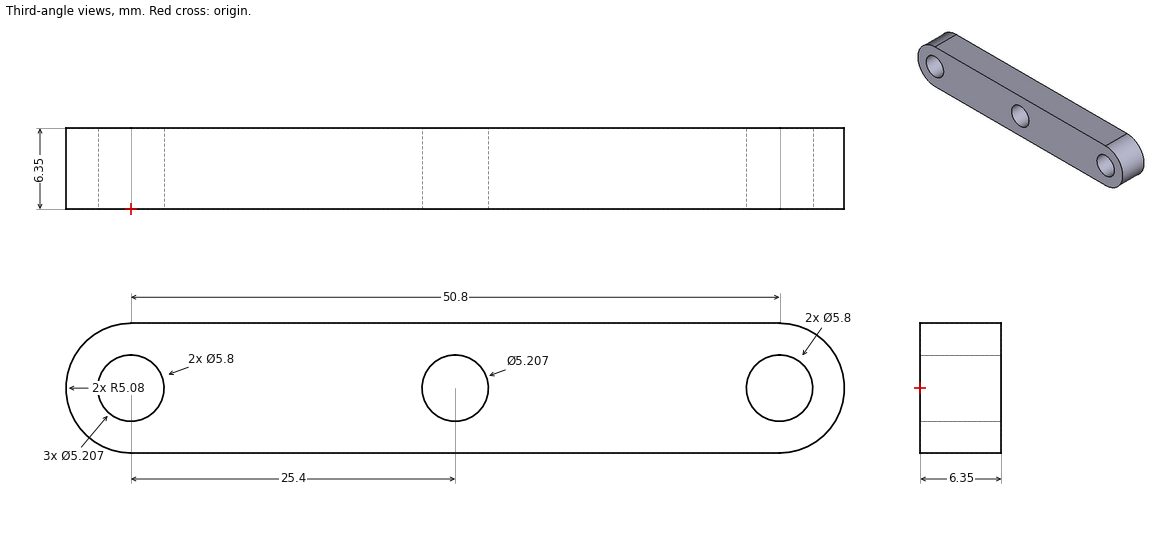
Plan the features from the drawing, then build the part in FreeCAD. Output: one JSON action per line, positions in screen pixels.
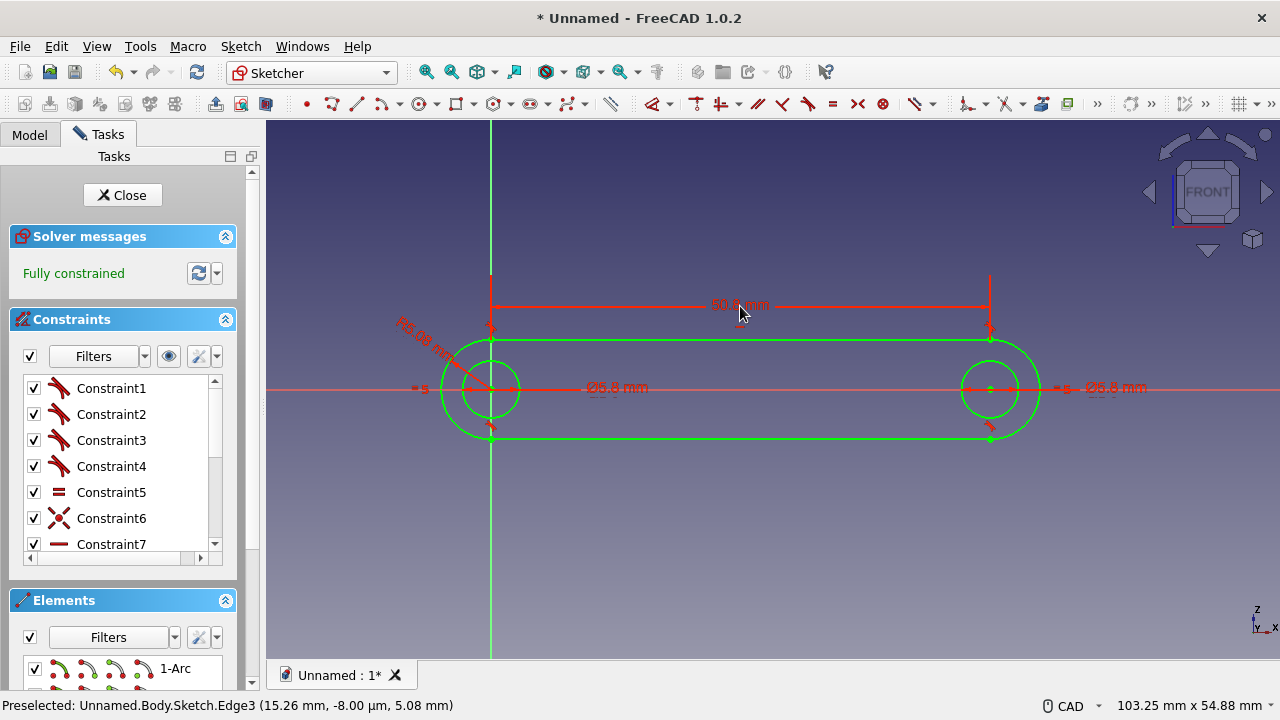
{"action": "left_click", "coordinate": [123, 195]}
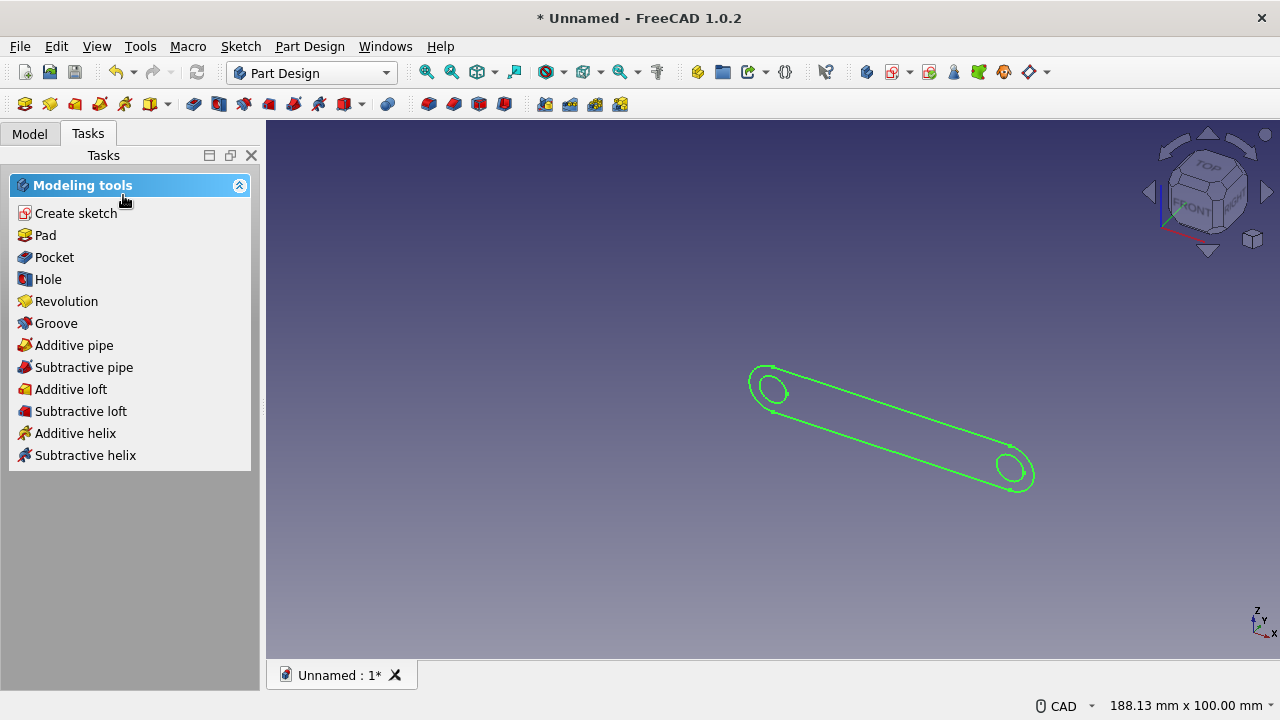
{"action": "left_click", "coordinate": [25, 104]}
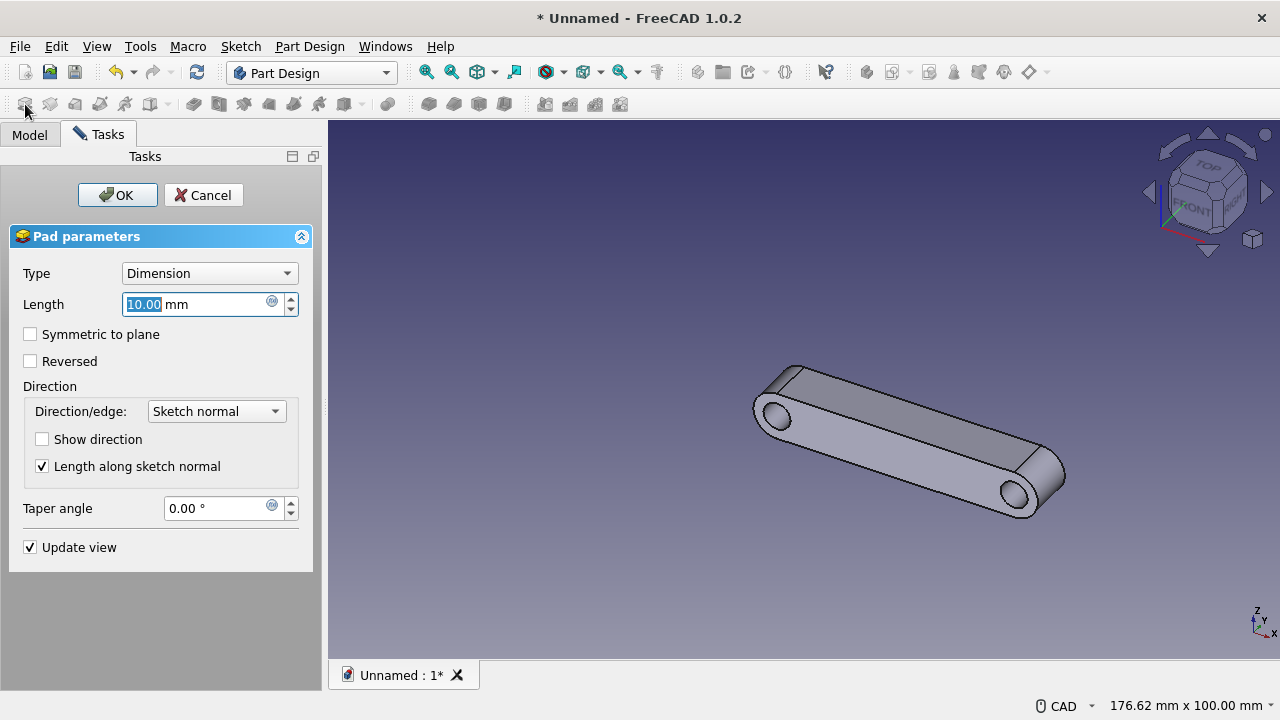
{"action": "type", "text": "6.35"}
{"action": "key", "text": "Tab"}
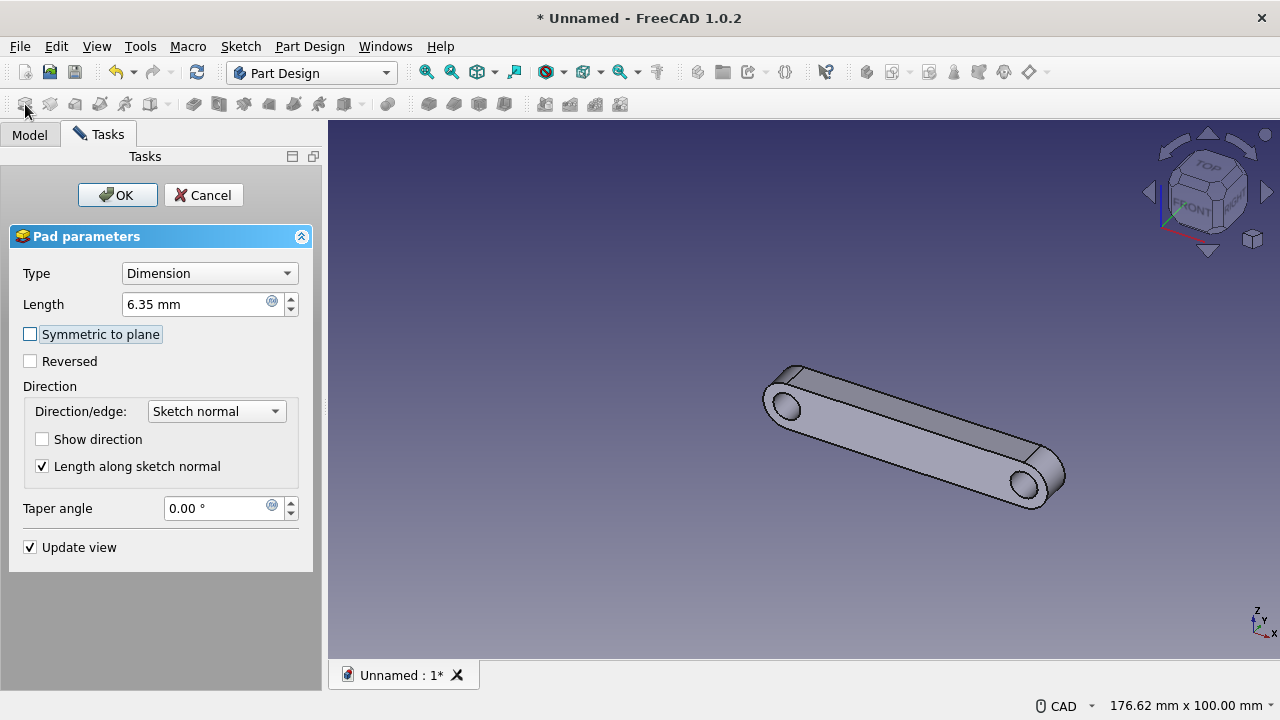
{"action": "left_click", "coordinate": [31, 361]}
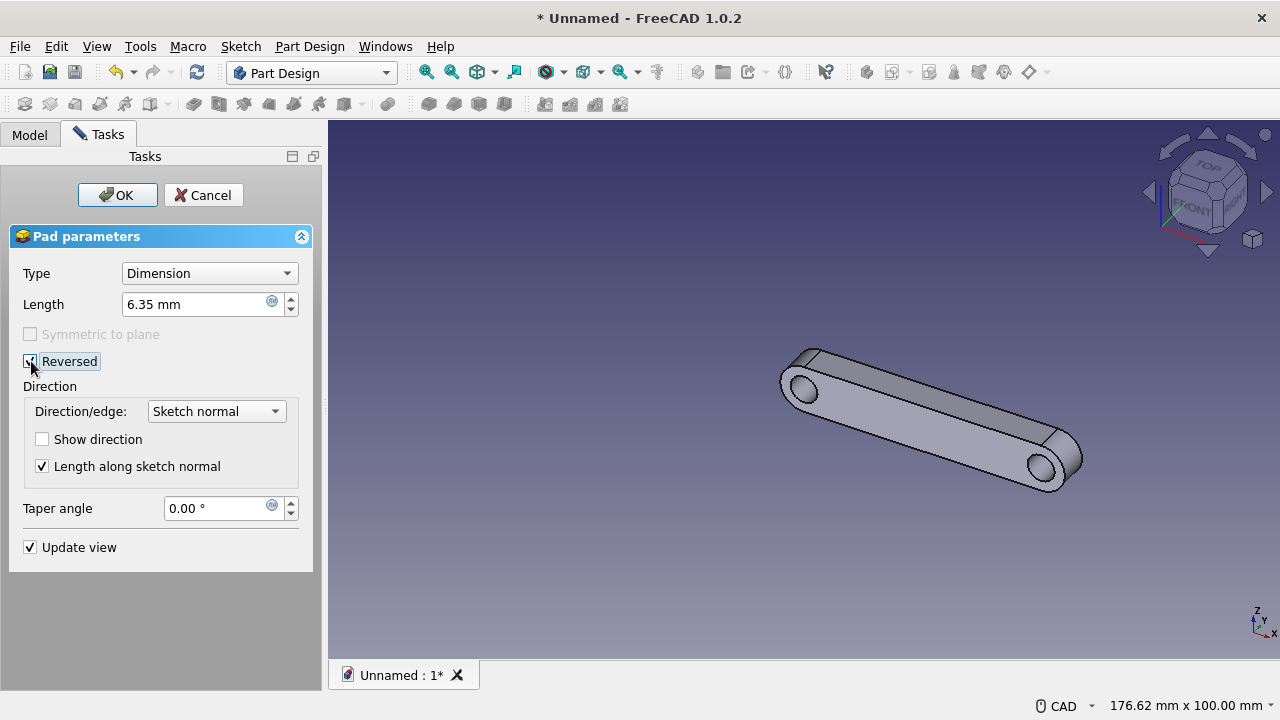
{"action": "left_click", "coordinate": [118, 195]}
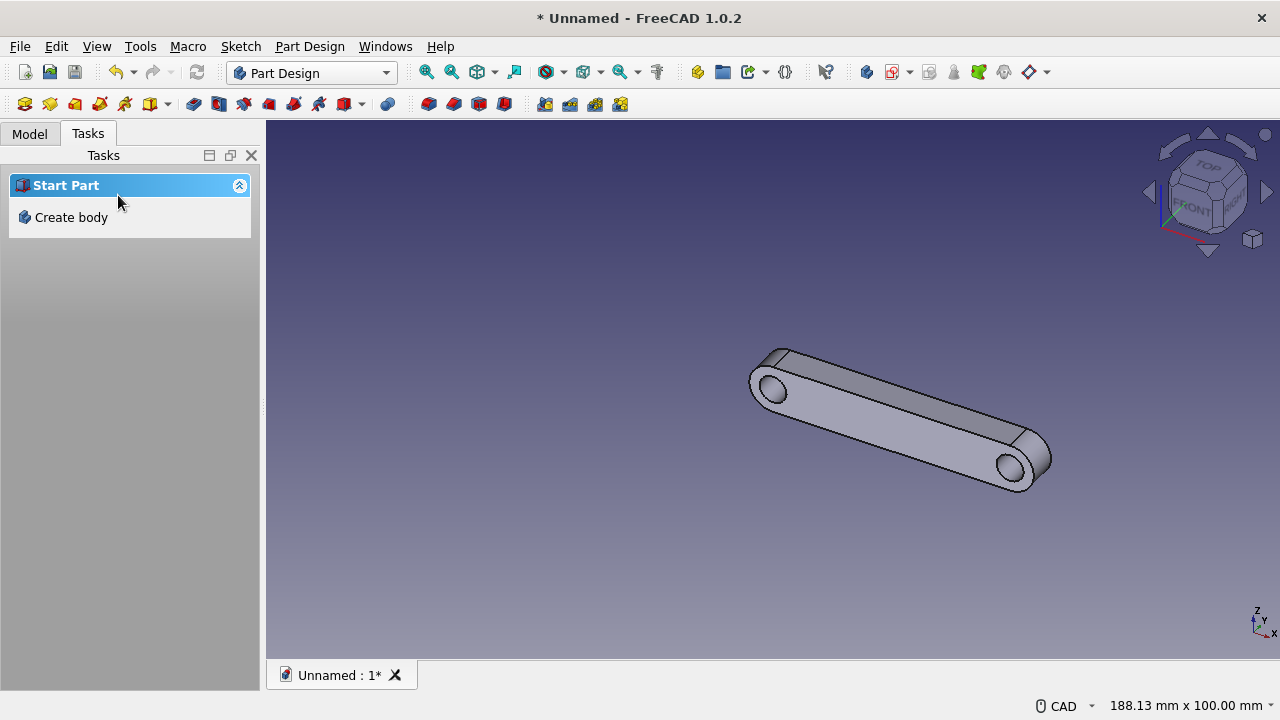
{"action": "left_click", "coordinate": [427, 72]}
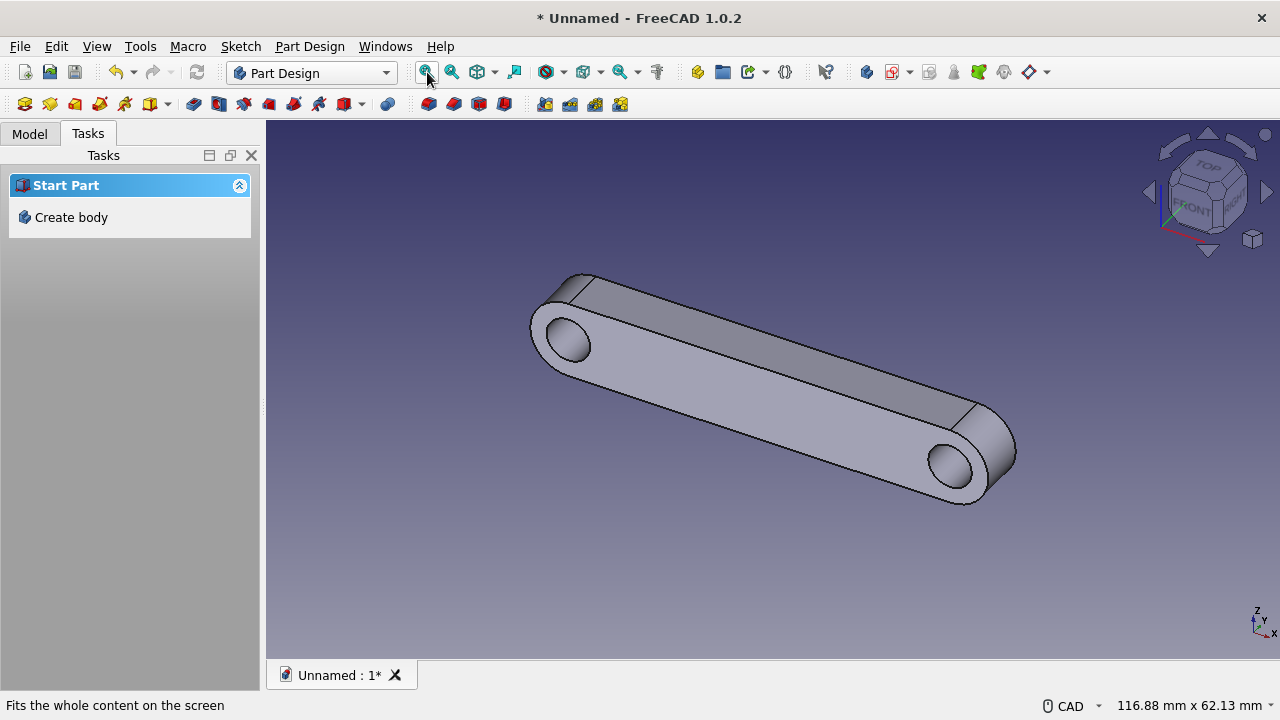
{"action": "left_click", "coordinate": [890, 446]}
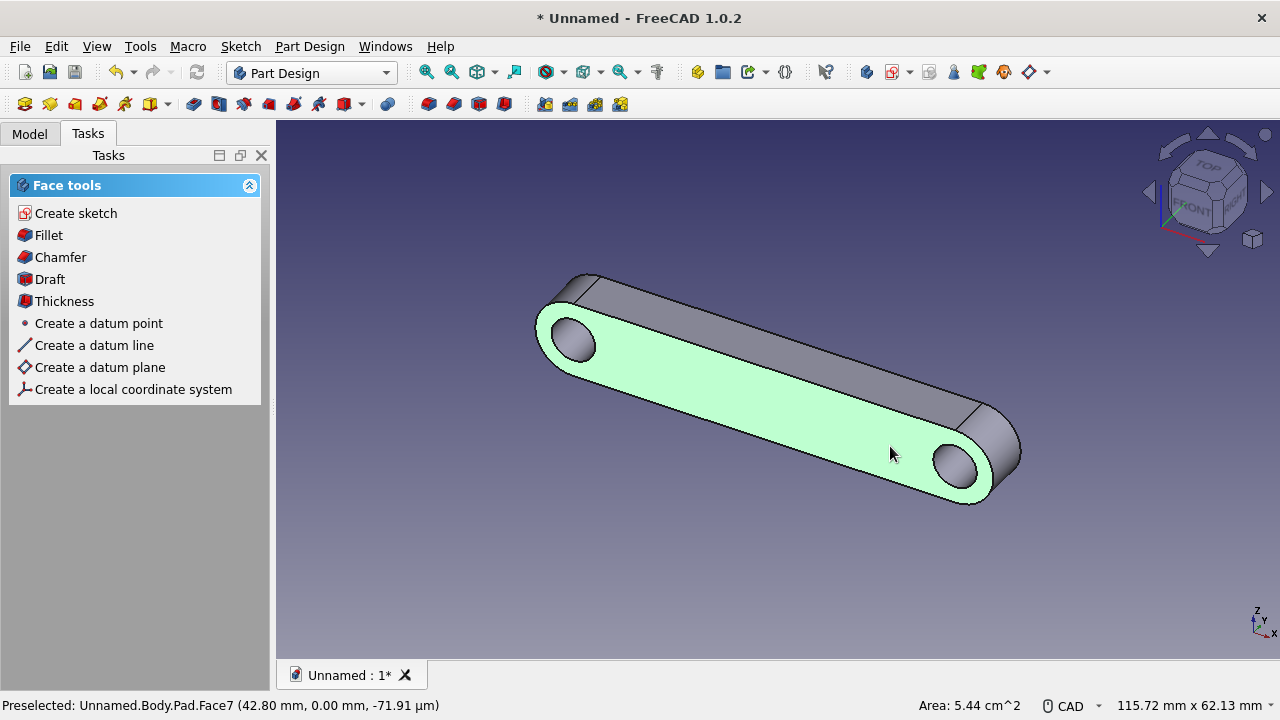
{"action": "left_click", "coordinate": [892, 72]}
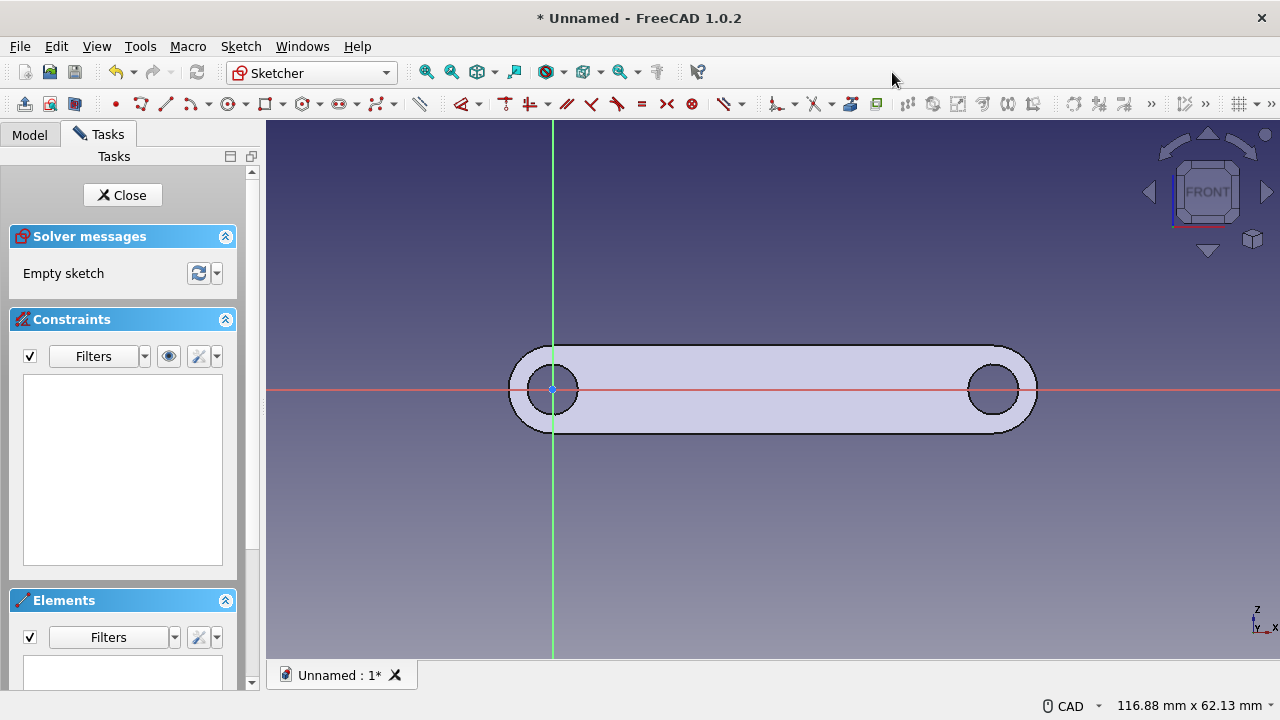
{"action": "key", "text": "g c"}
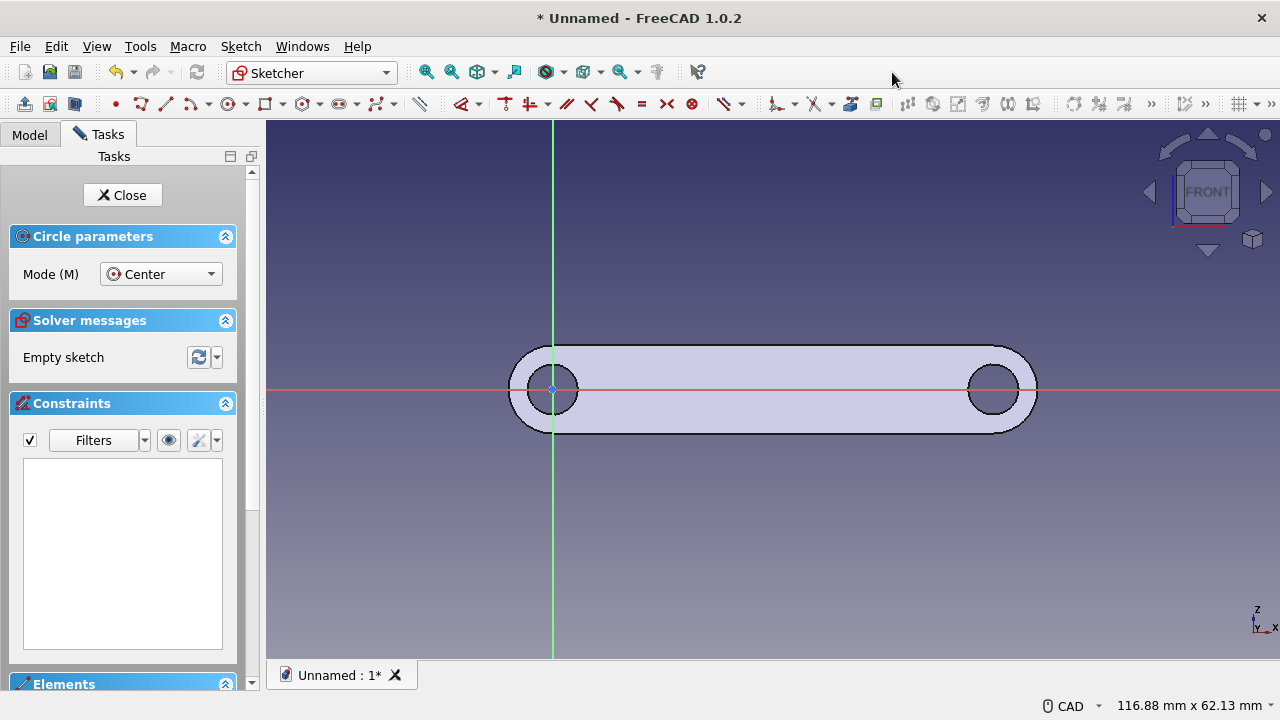
{"action": "left_click", "coordinate": [553, 390]}
{"action": "mouse_move", "coordinate": [570, 372]}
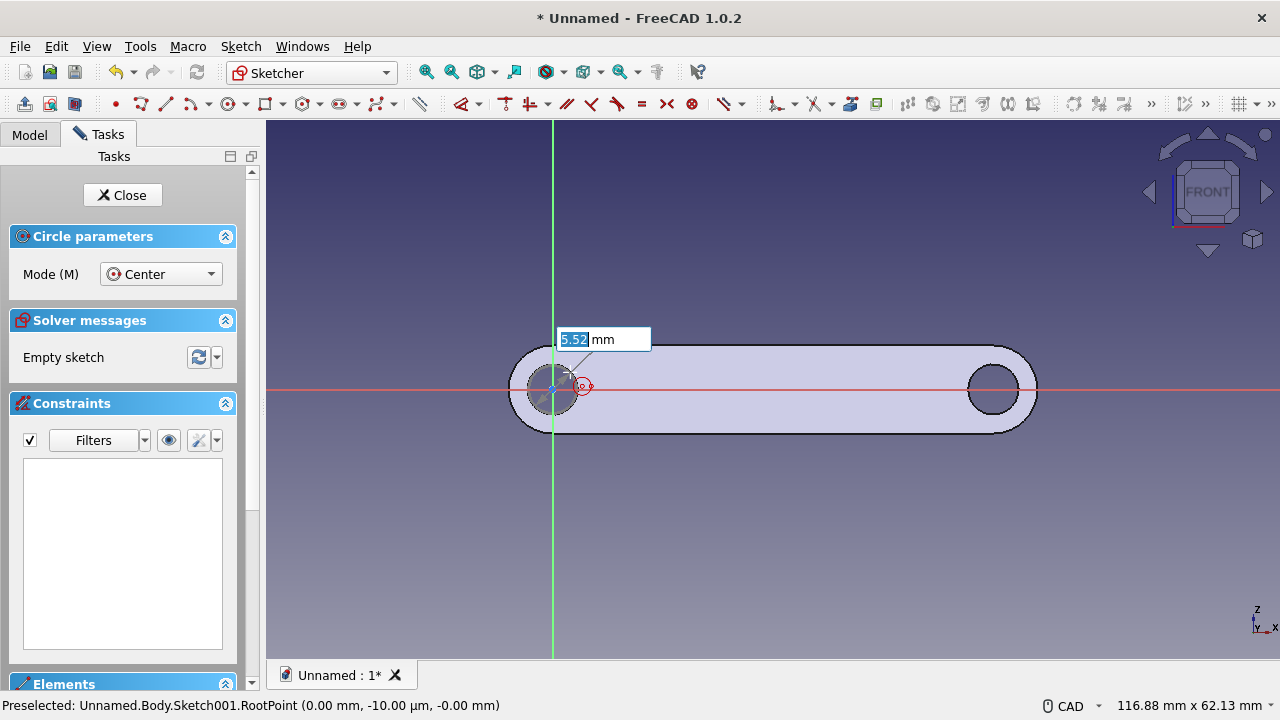
{"action": "type", "text": "5.8"}
{"action": "key", "text": "Return"}